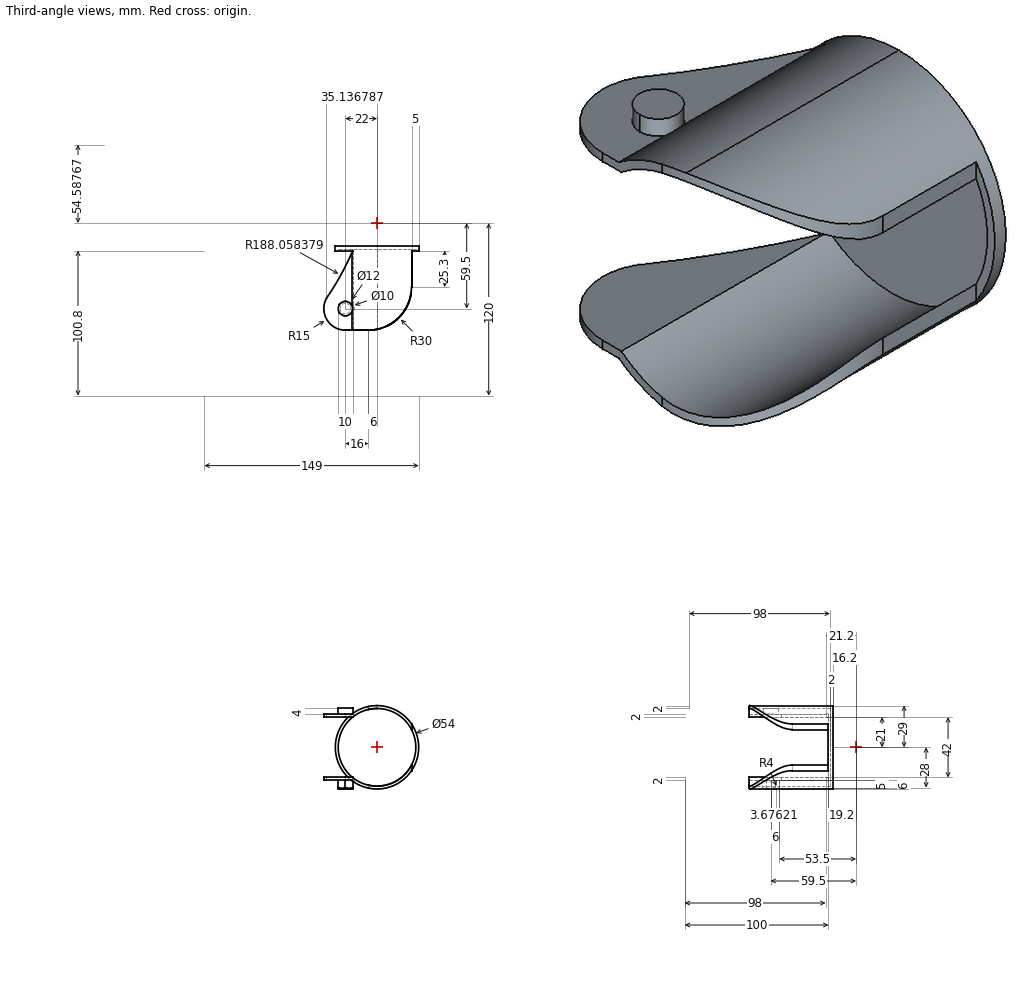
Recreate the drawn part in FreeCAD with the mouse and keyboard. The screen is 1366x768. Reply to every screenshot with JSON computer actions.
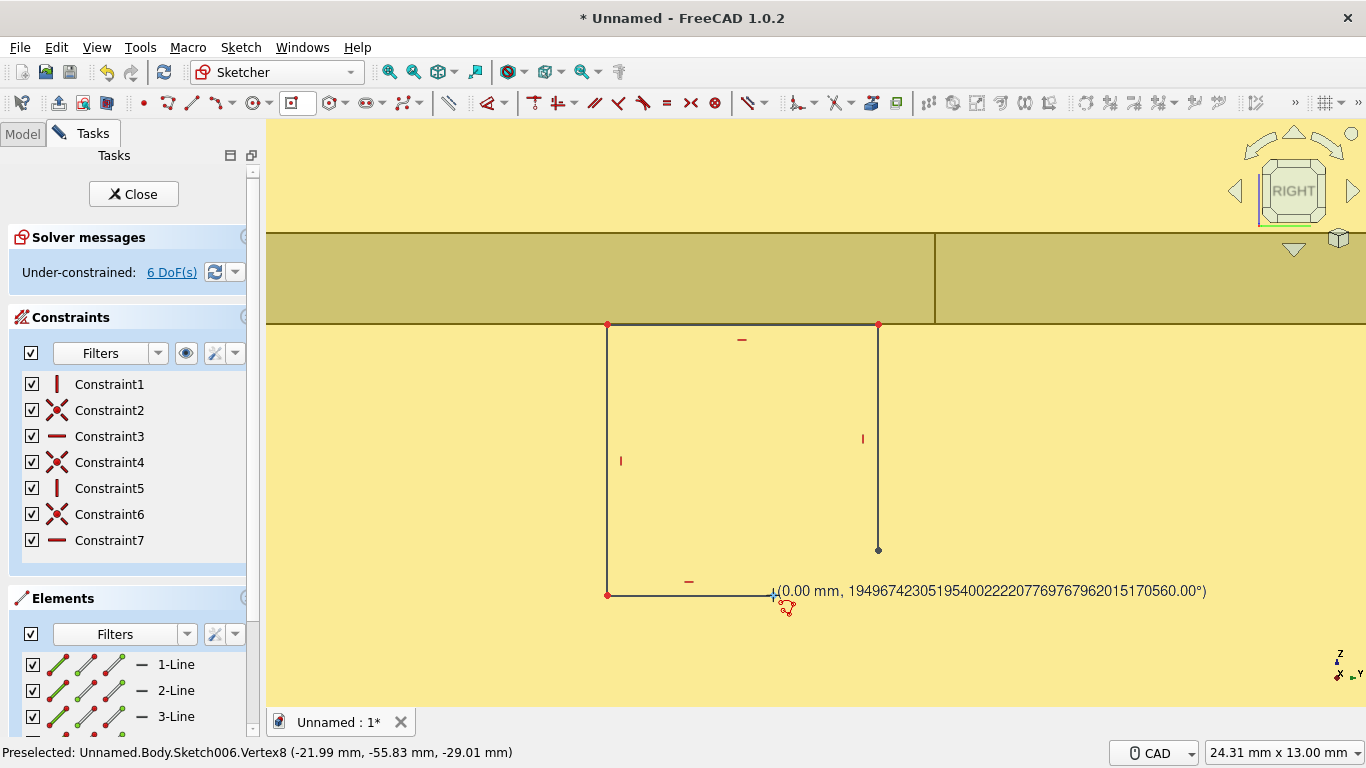
{"action": "left_click", "coordinate": [216, 104]}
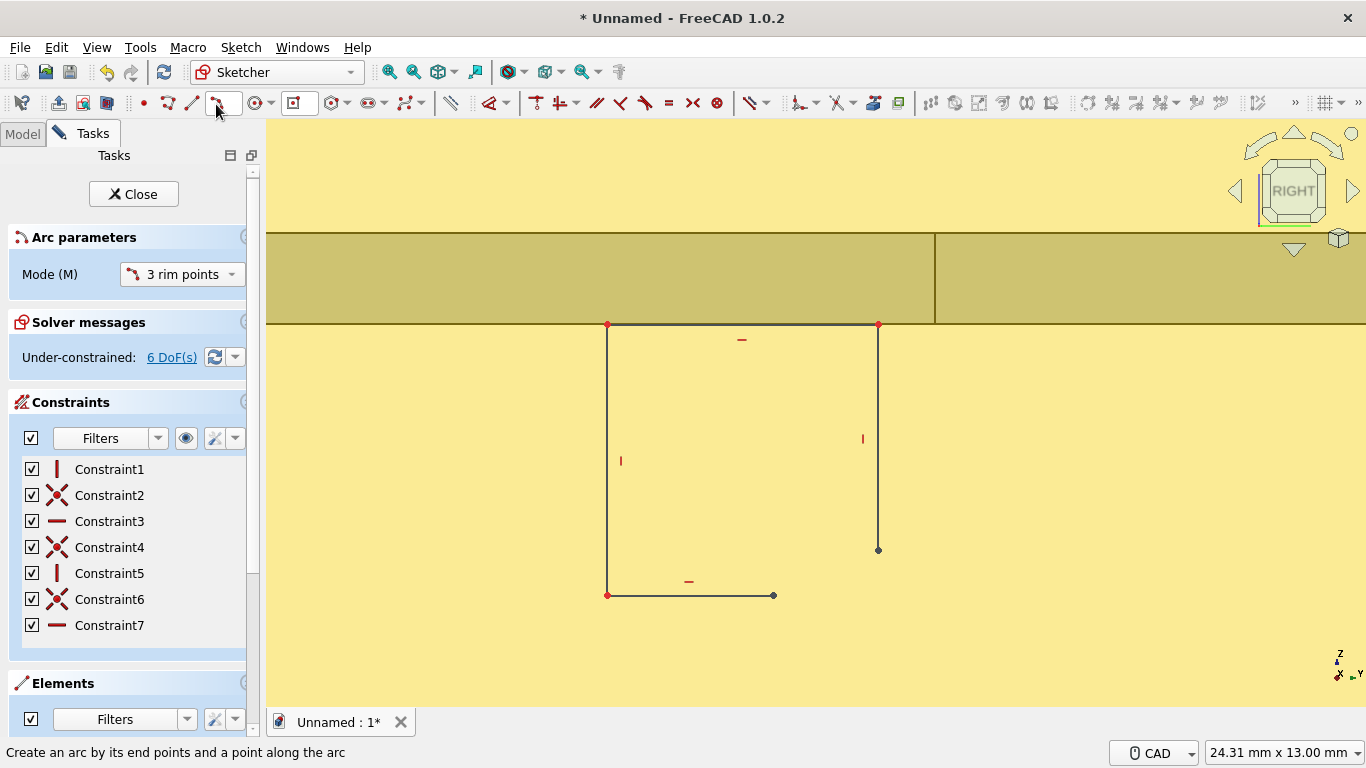
{"action": "left_click", "coordinate": [773, 596]}
{"action": "left_click", "coordinate": [878, 551]}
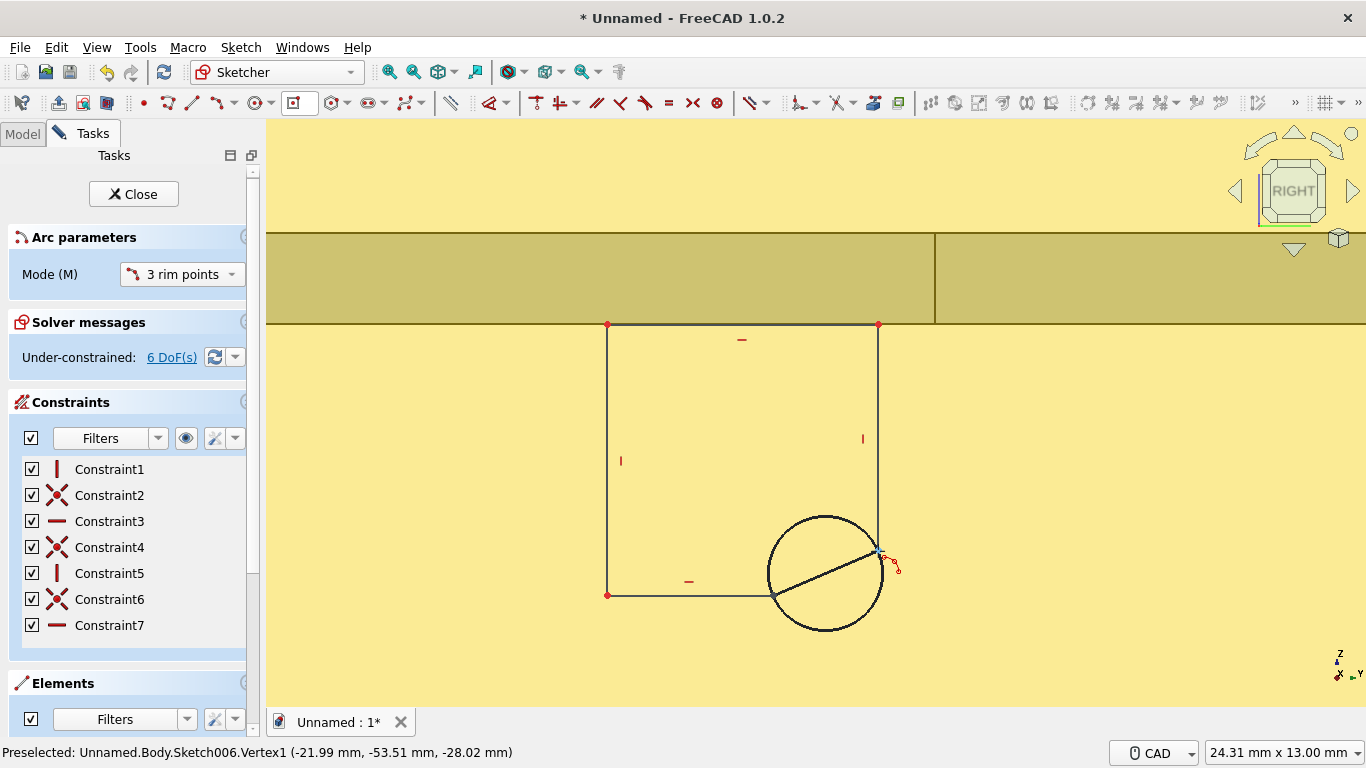
{"action": "scroll", "coordinate": [830, 581], "scroll_direction": "up", "scroll_amount": 3}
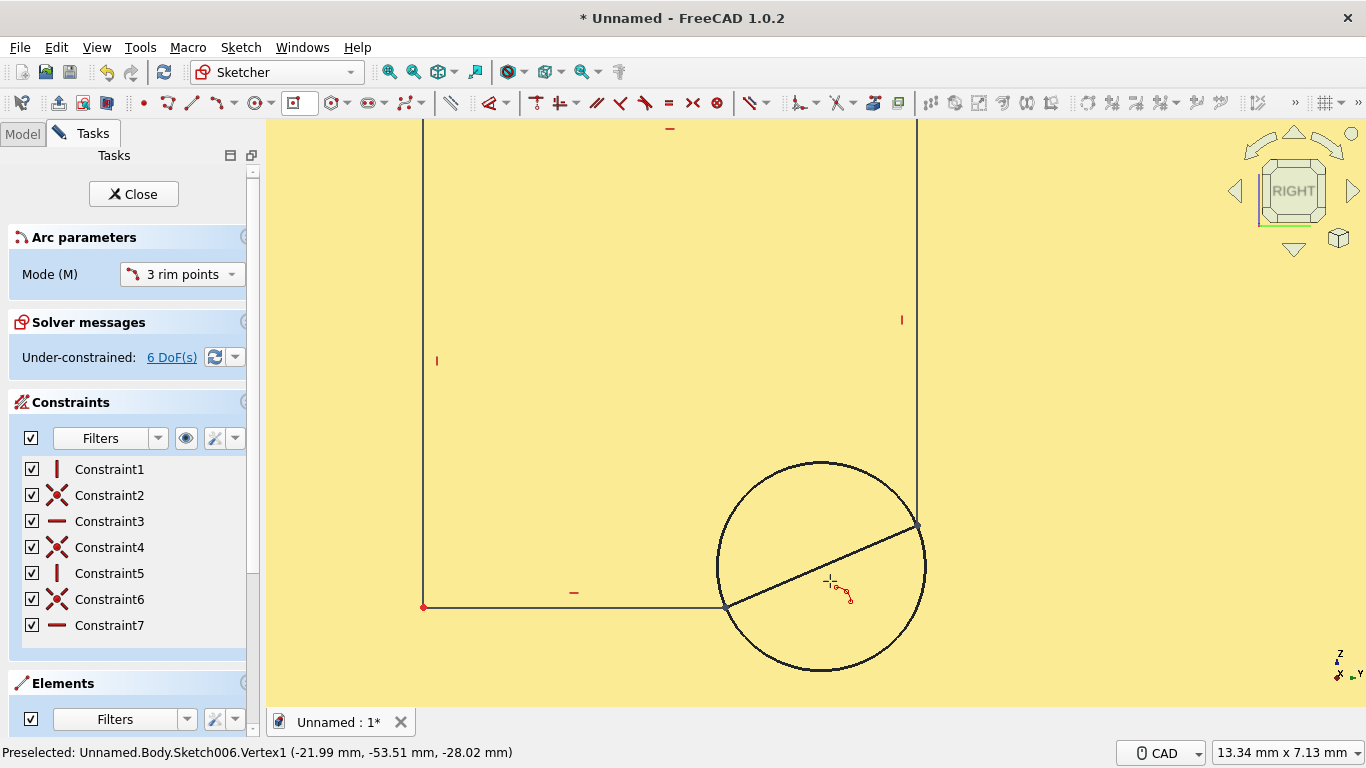
{"action": "left_click", "coordinate": [829, 581]}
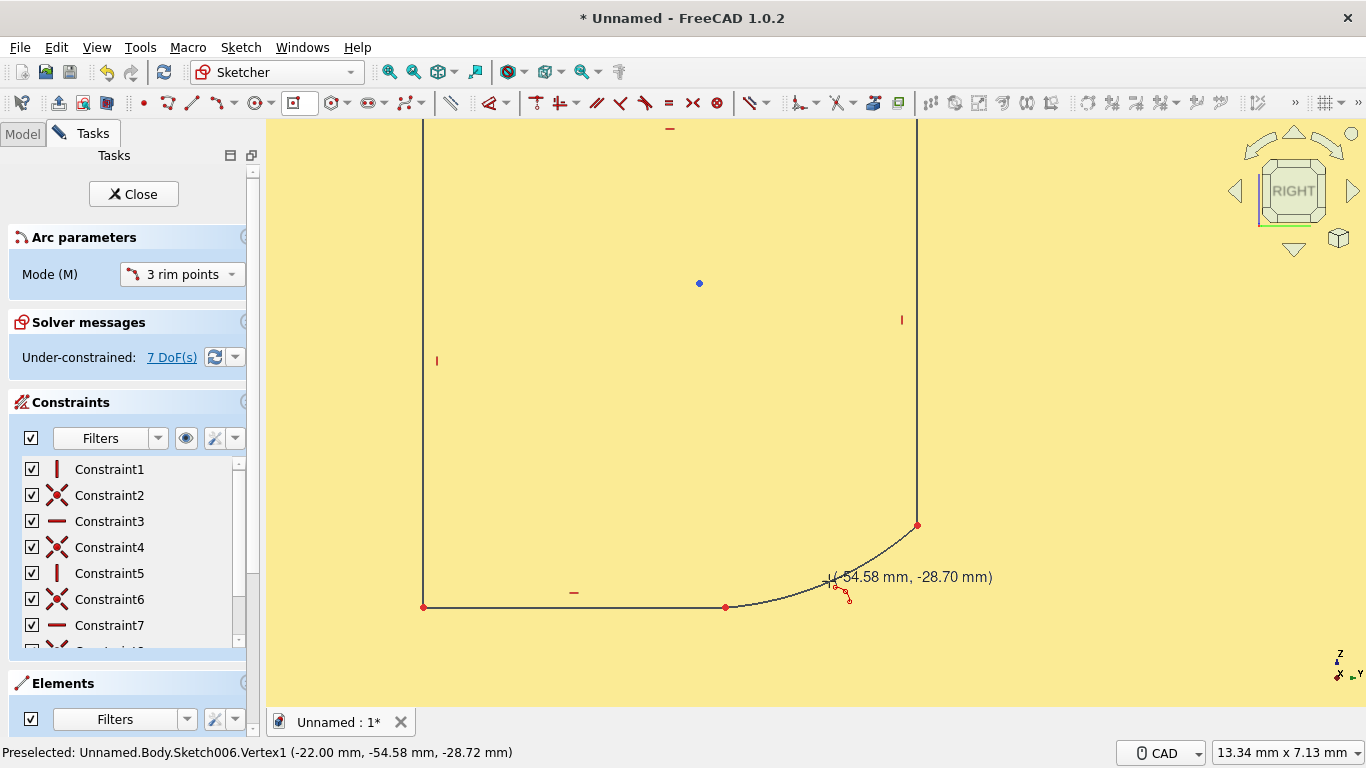
{"action": "key", "text": "g l"}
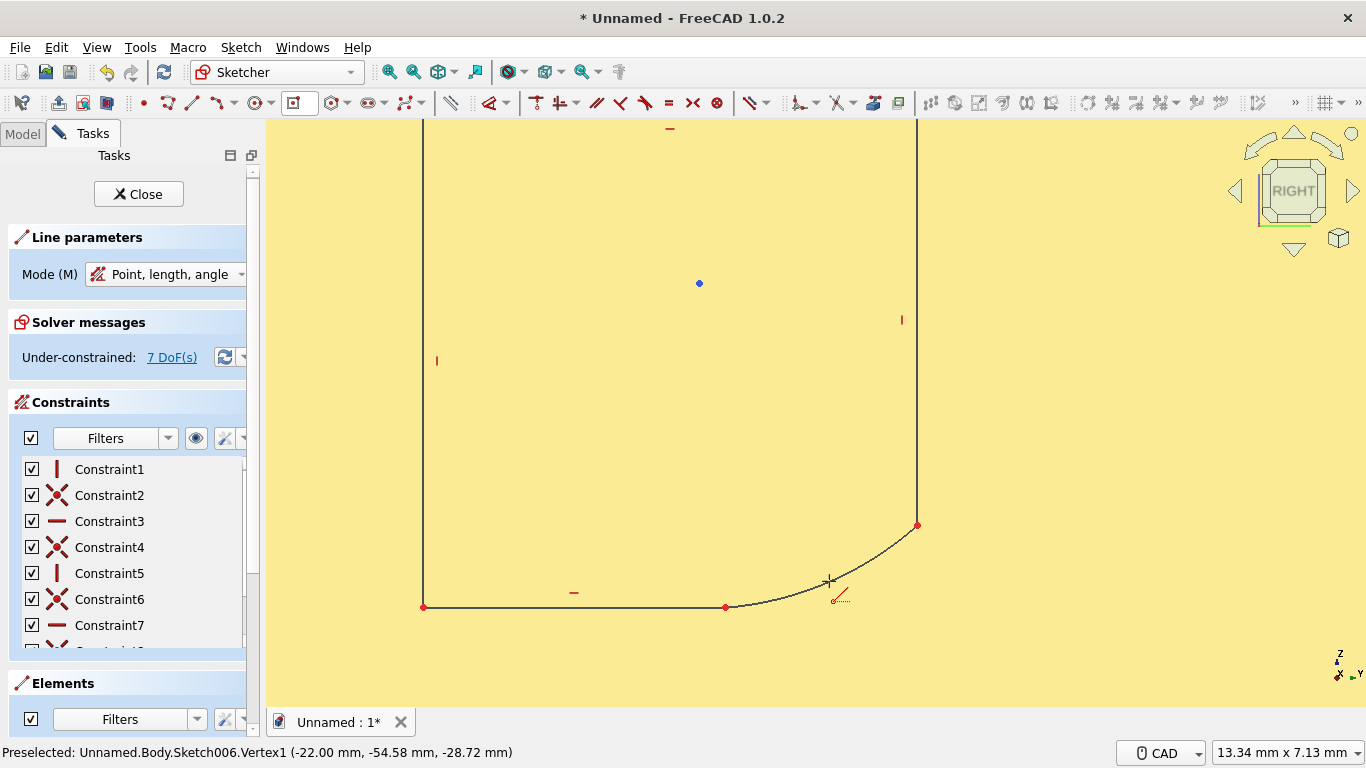
{"action": "scroll", "coordinate": [841, 599], "scroll_direction": "down", "scroll_amount": 3}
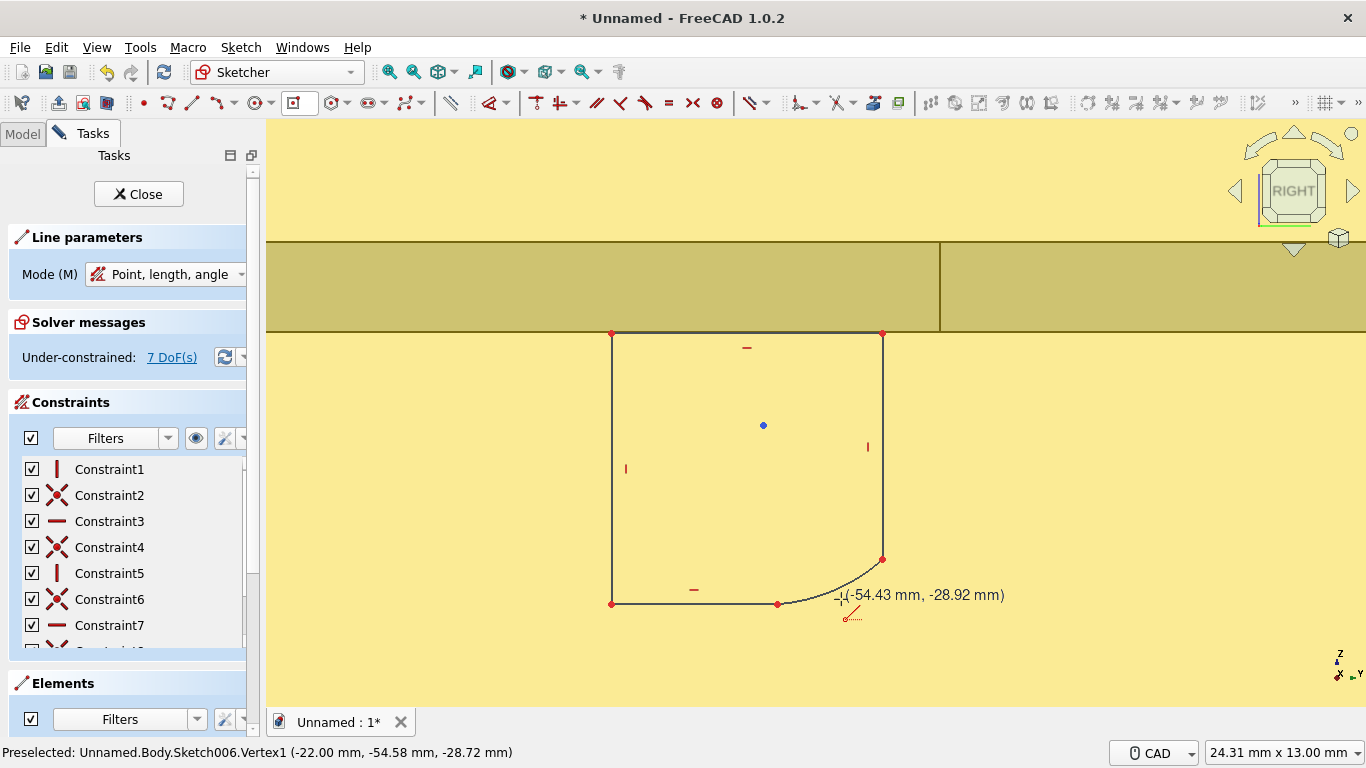
{"action": "left_click", "coordinate": [612, 305]}
{"action": "left_click", "coordinate": [612, 223]}
{"action": "key", "text": "Escape"}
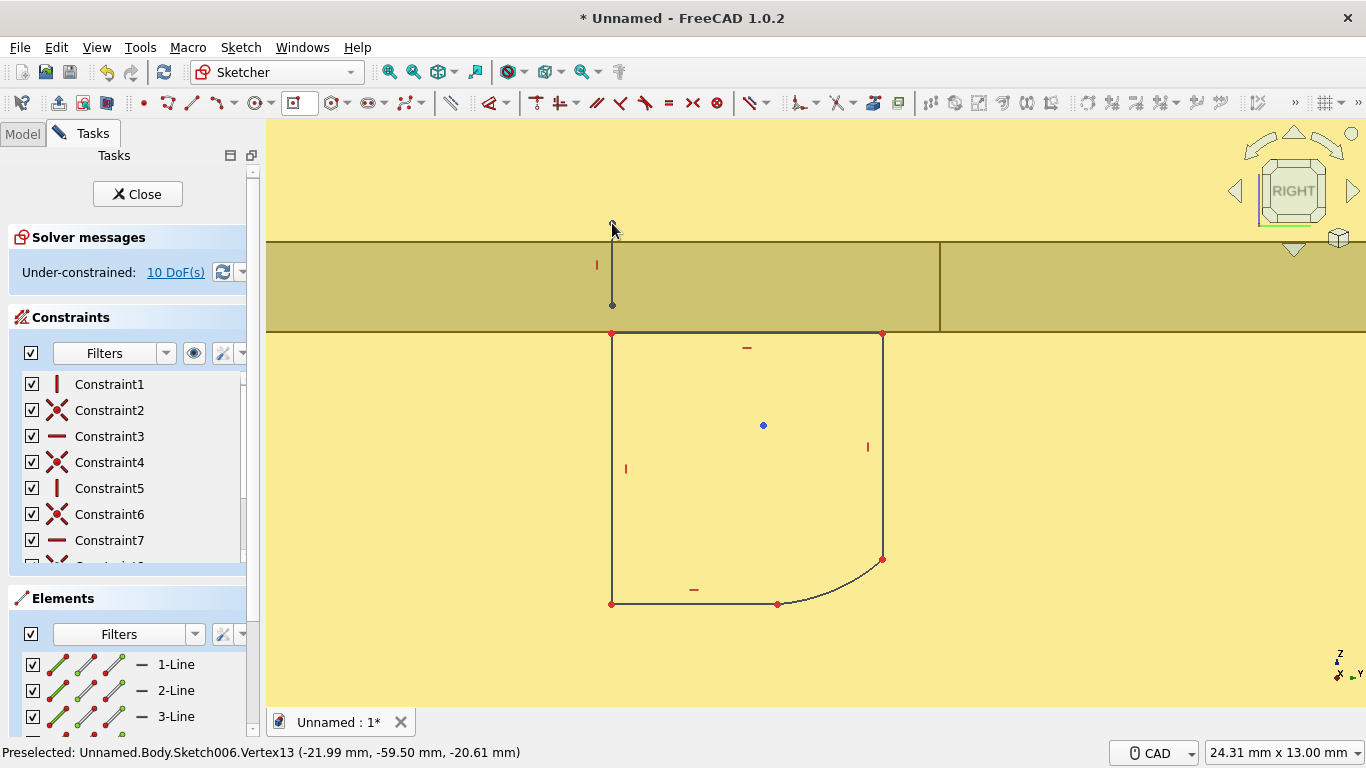
{"action": "left_click", "coordinate": [612, 281]}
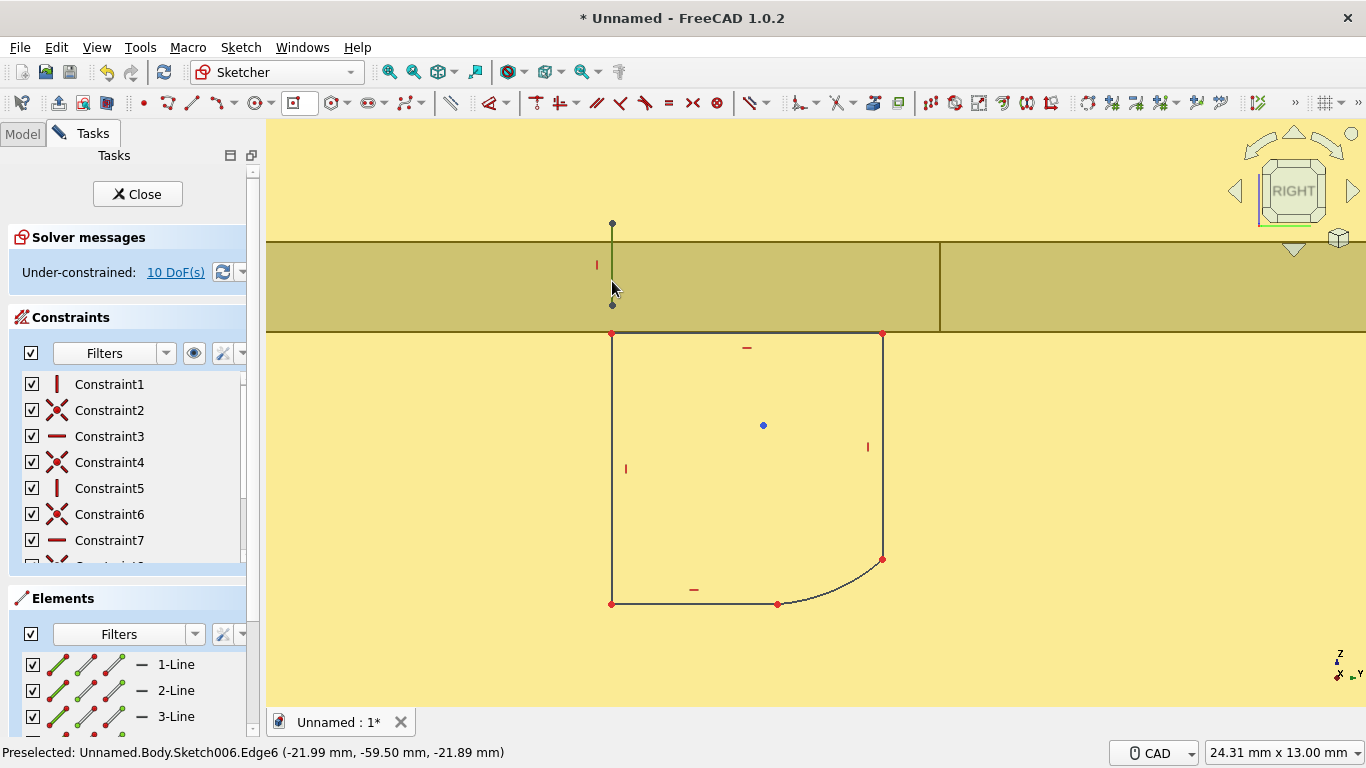
{"action": "key", "text": "g n"}